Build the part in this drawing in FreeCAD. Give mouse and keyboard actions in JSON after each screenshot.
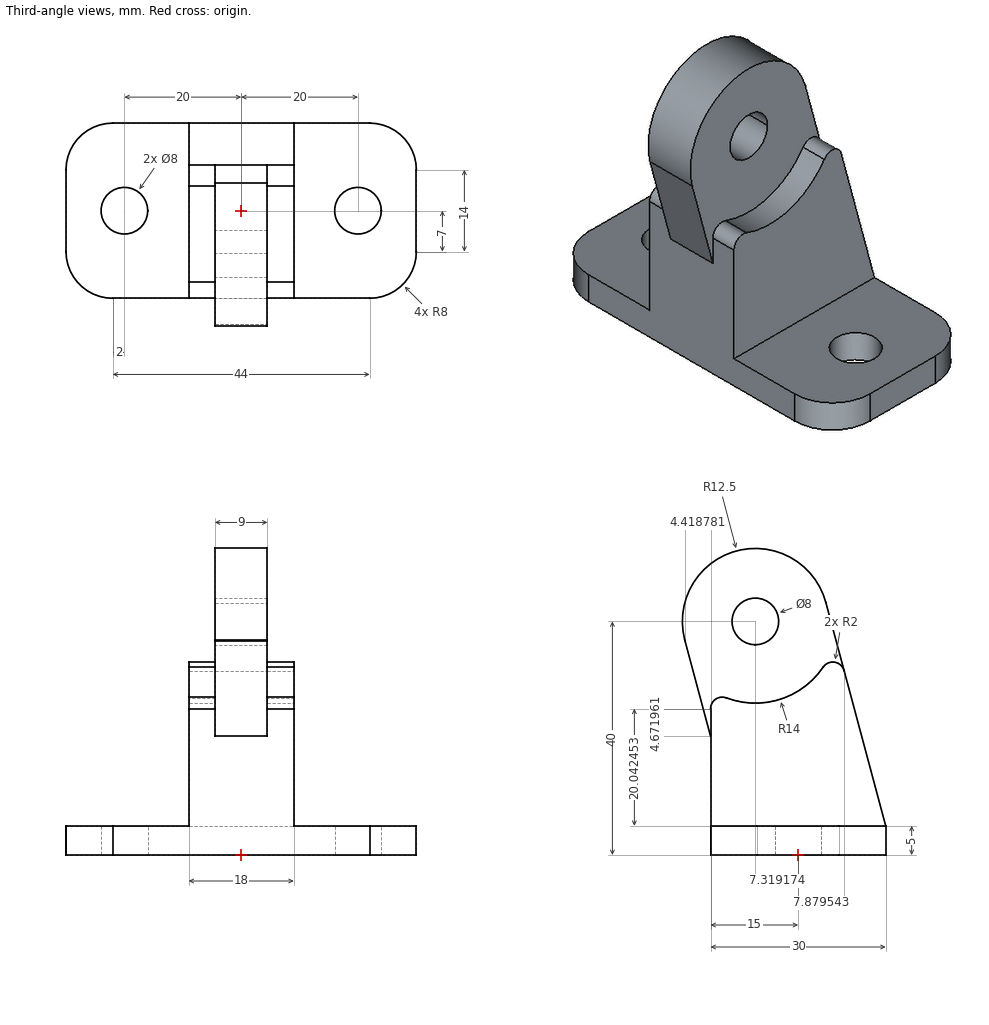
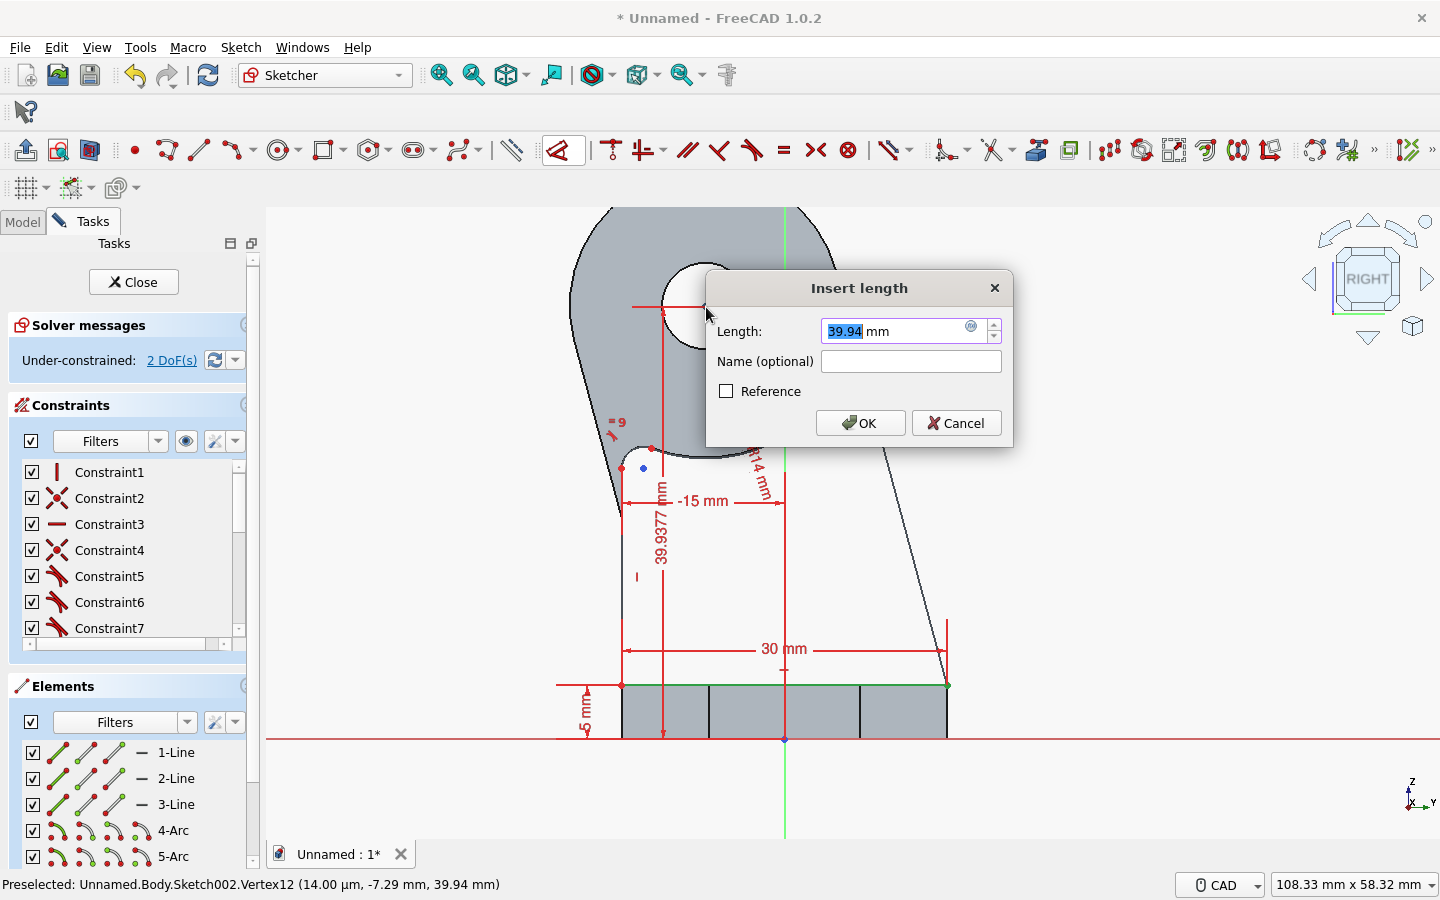
{"action": "type", "text": "40"}
{"action": "key", "text": "Return"}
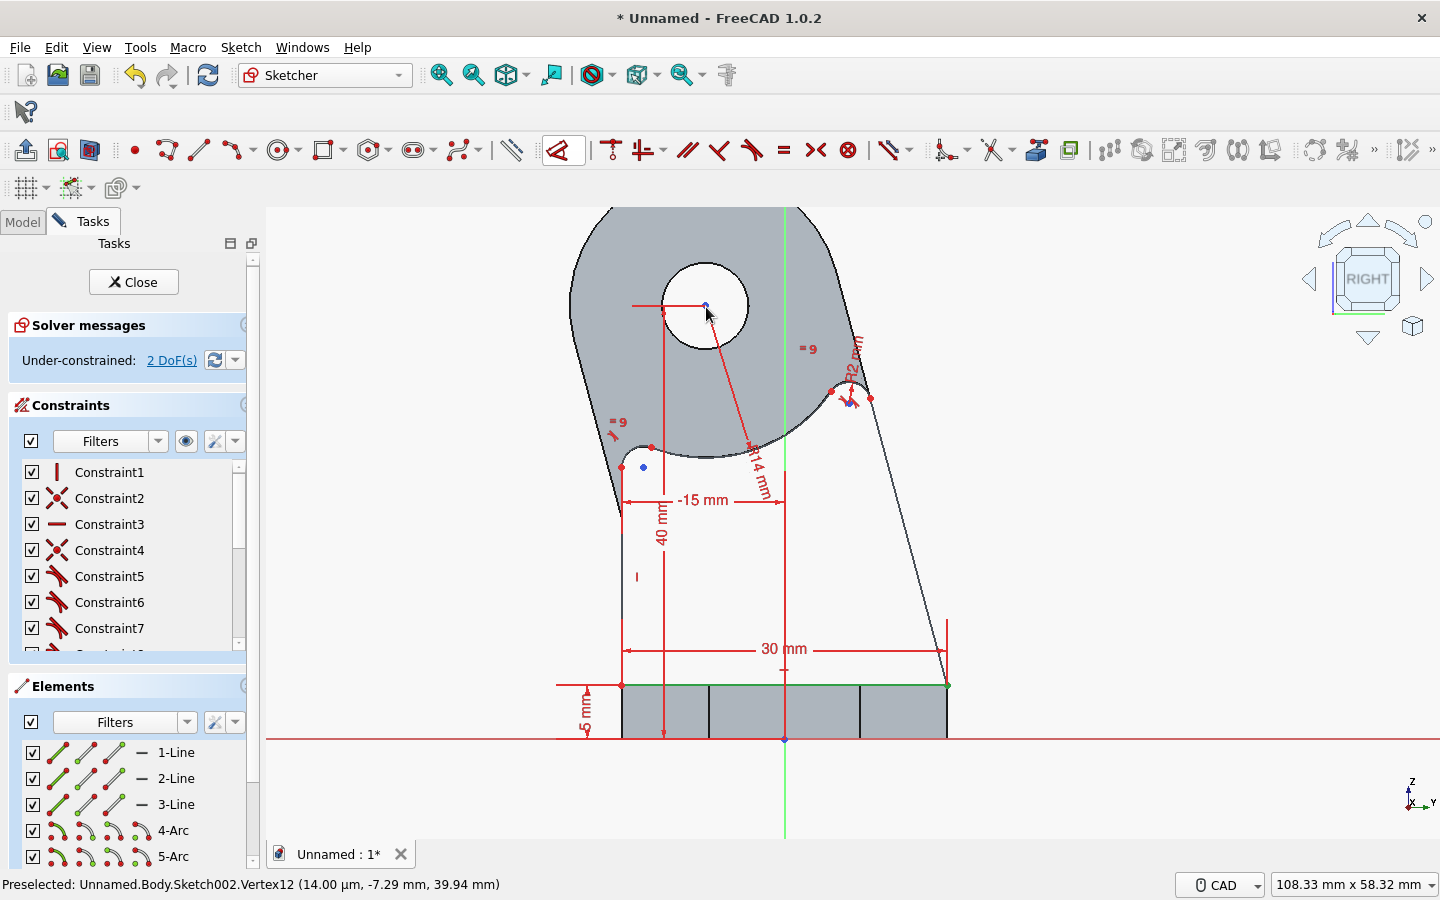
{"action": "left_click", "coordinate": [622, 533]}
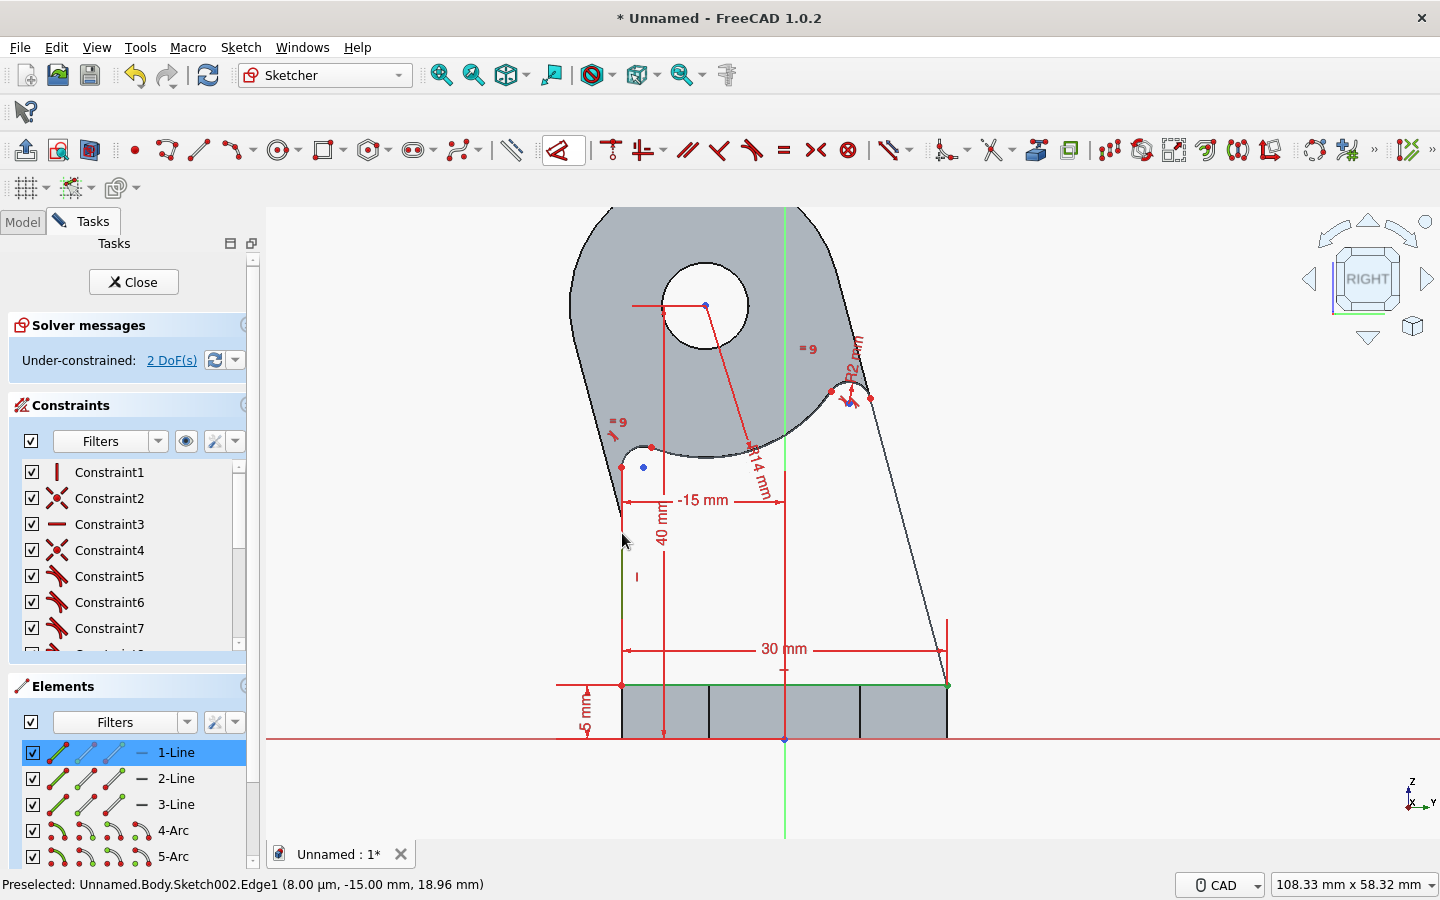
{"action": "key", "text": "i"}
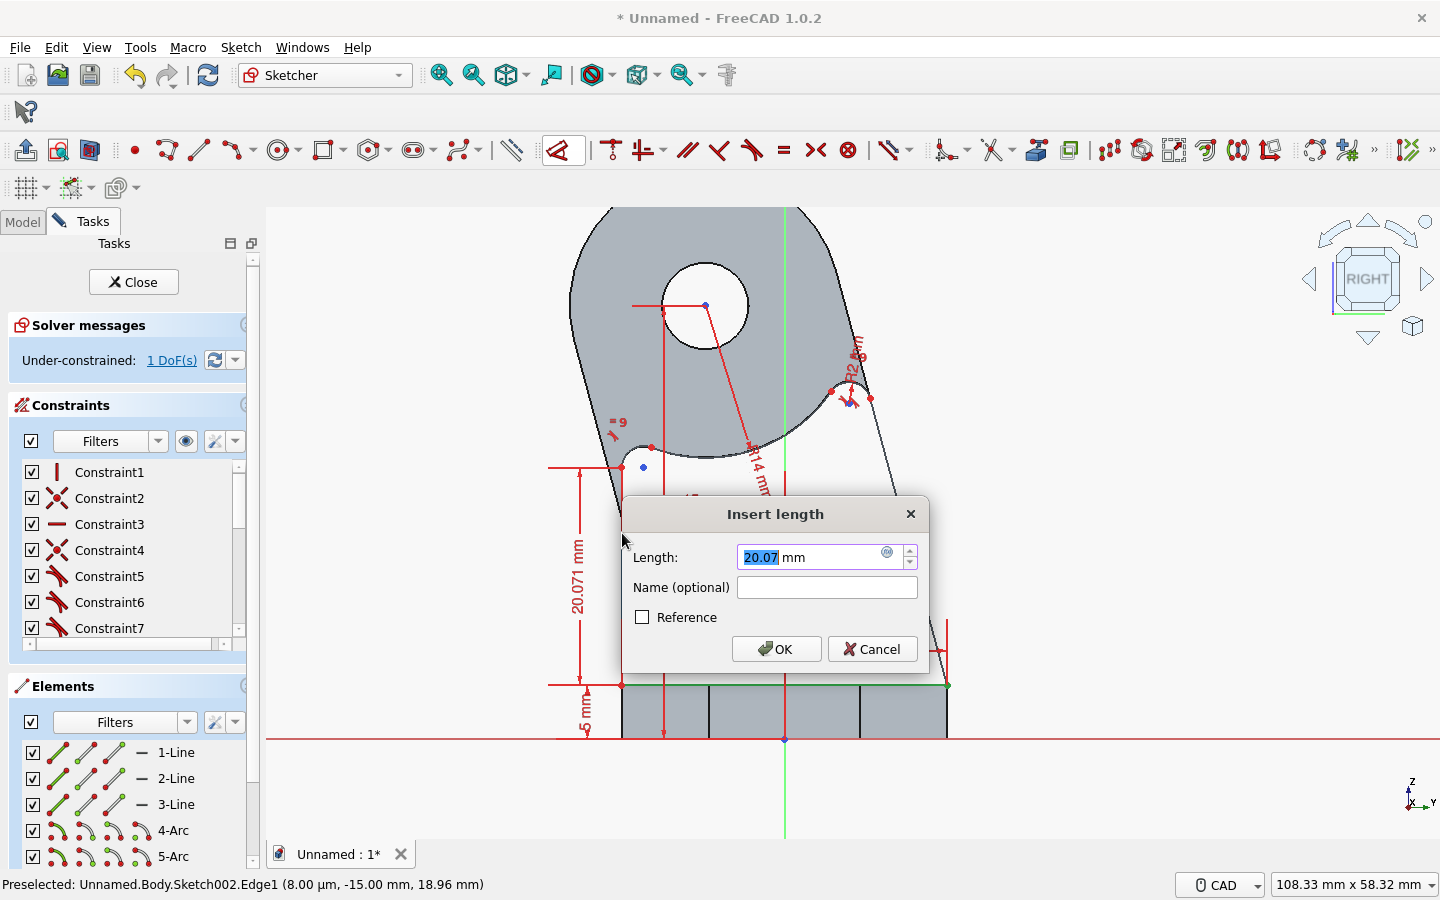
{"action": "type", "text": "20.042453"}
{"action": "key", "text": "Return"}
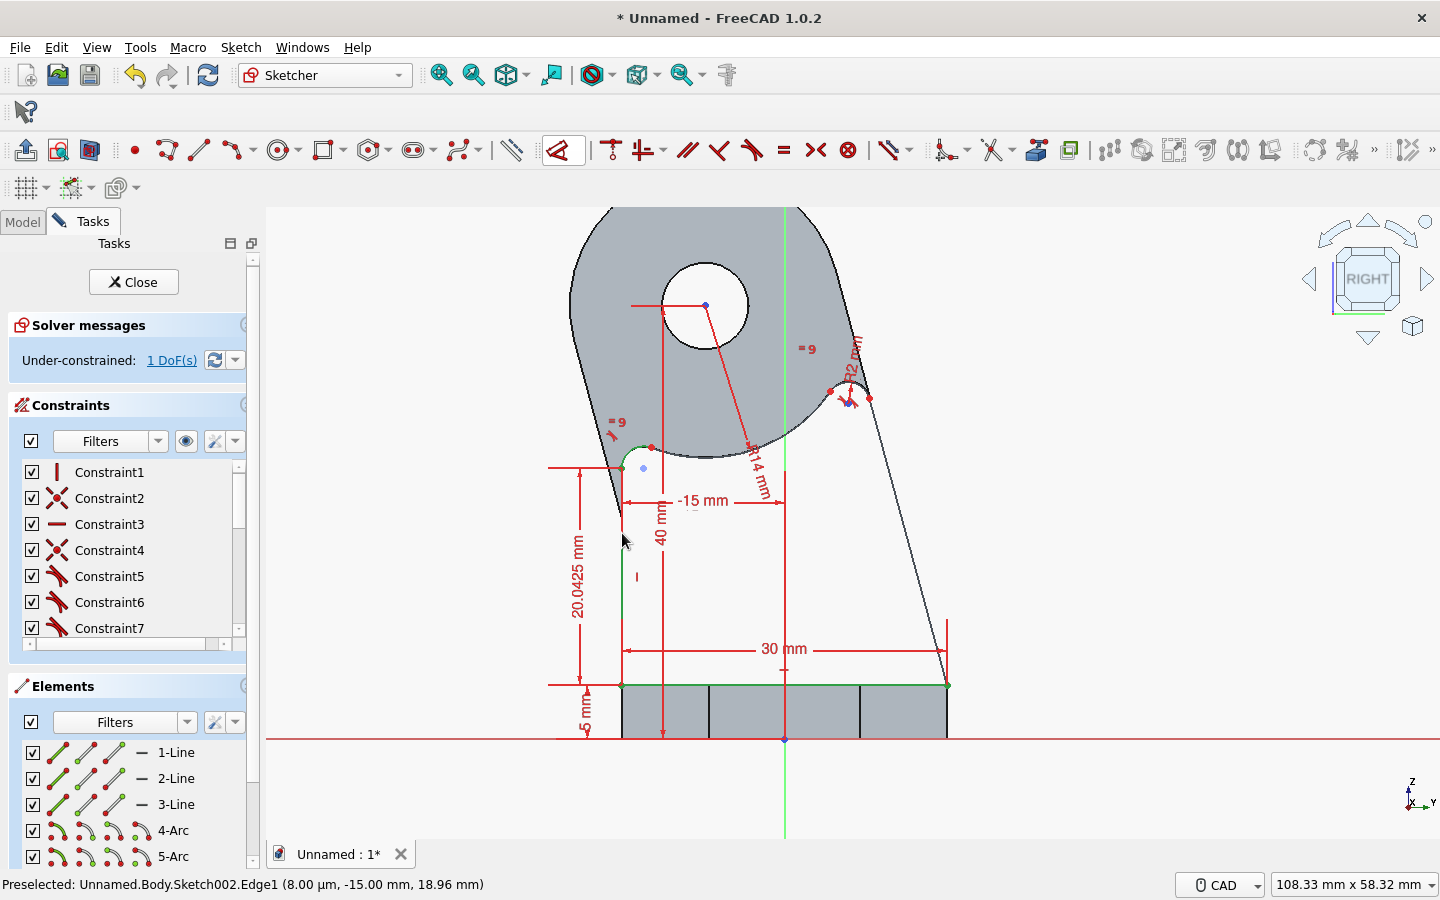
{"action": "left_click", "coordinate": [869, 398]}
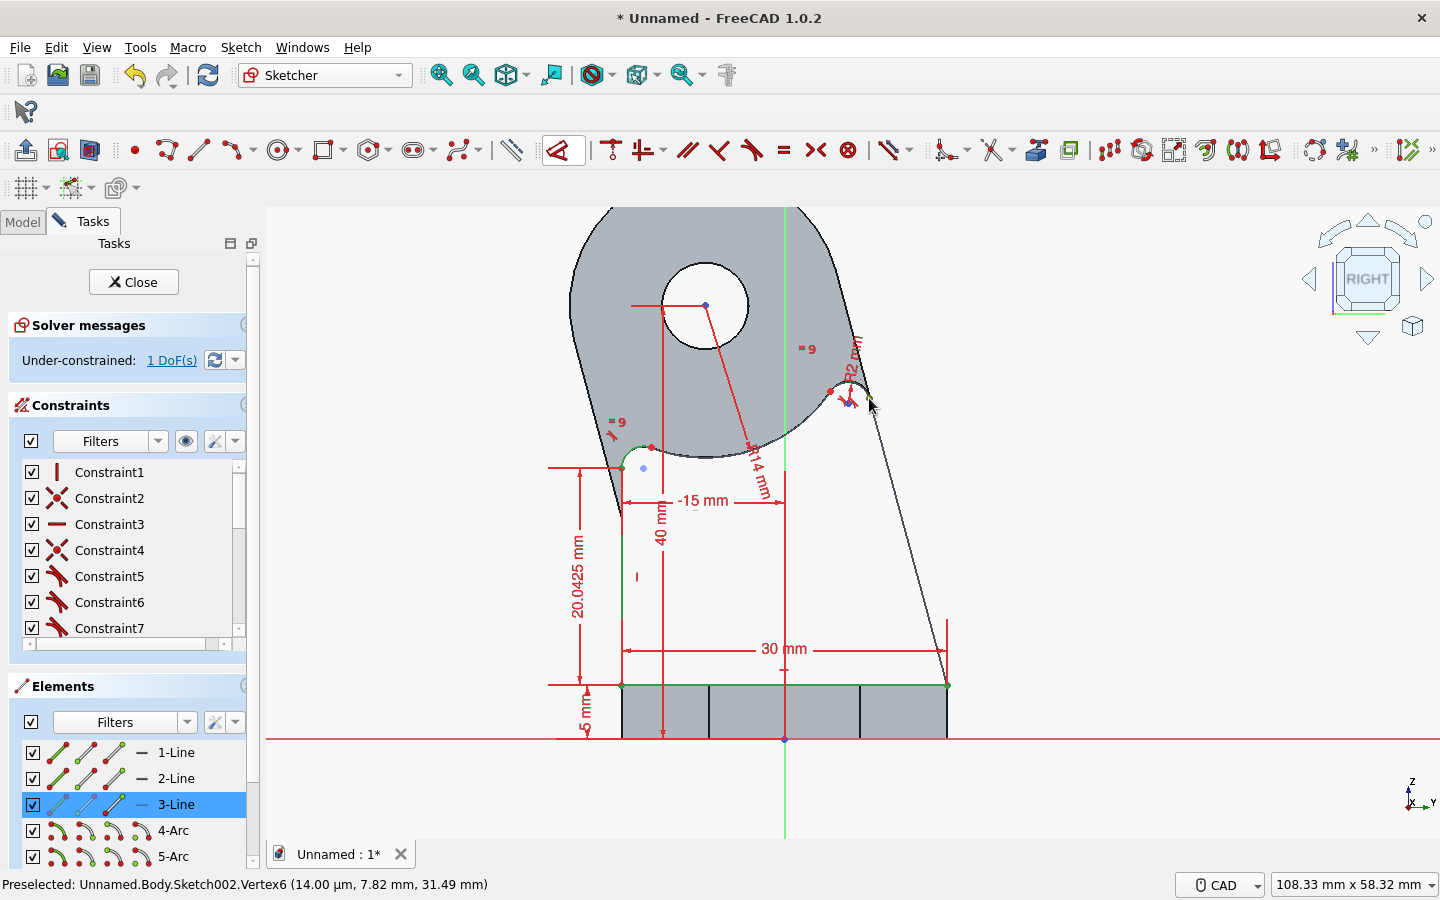
{"action": "key", "text": "l"}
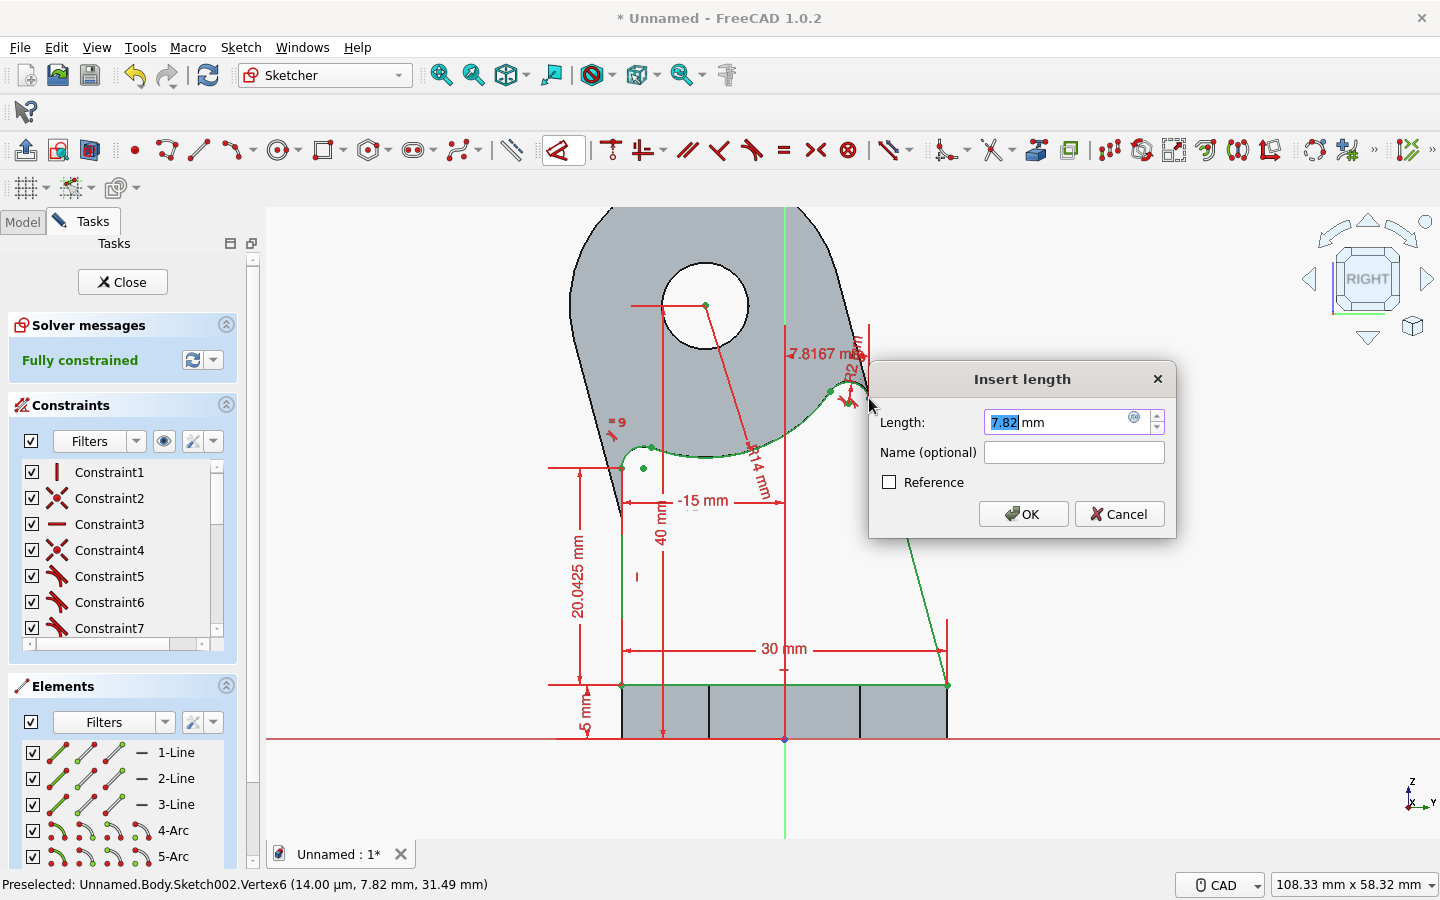
{"action": "type", "text": "7.879543"}
{"action": "key", "text": "Return"}